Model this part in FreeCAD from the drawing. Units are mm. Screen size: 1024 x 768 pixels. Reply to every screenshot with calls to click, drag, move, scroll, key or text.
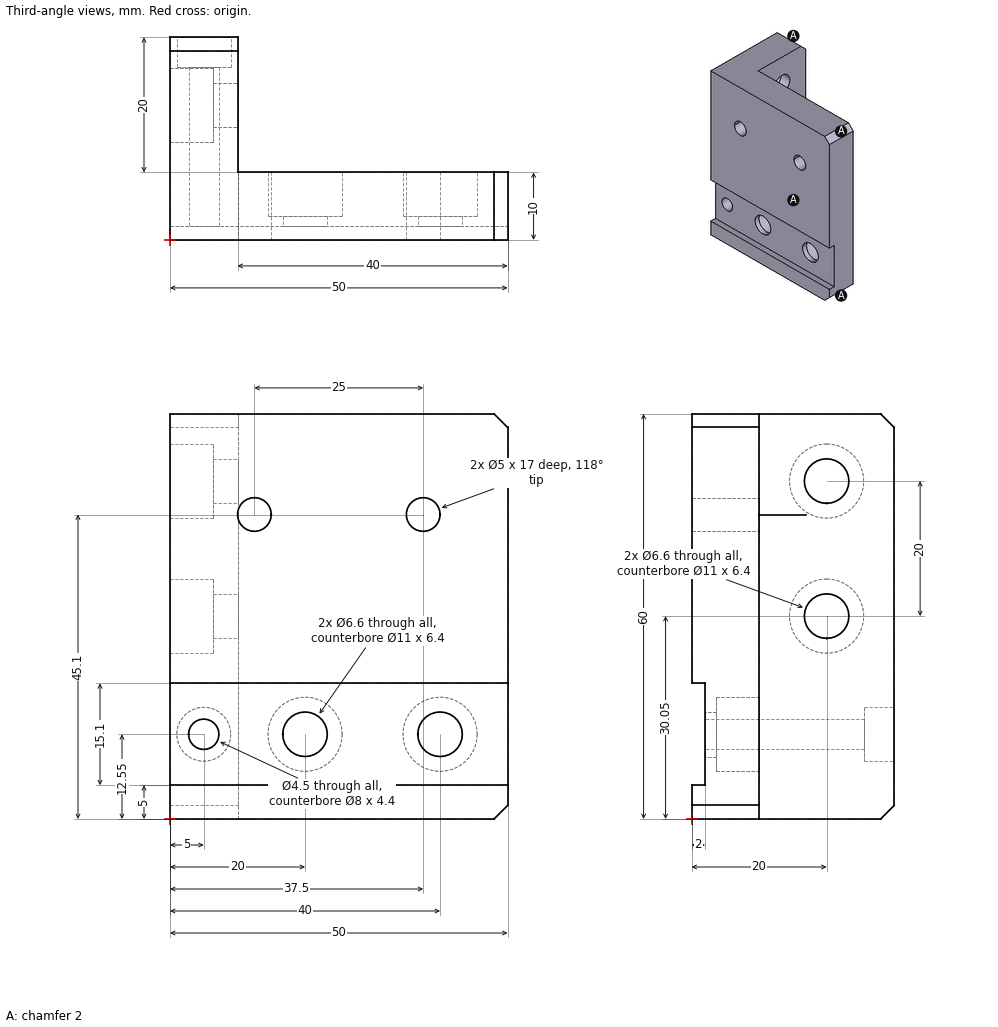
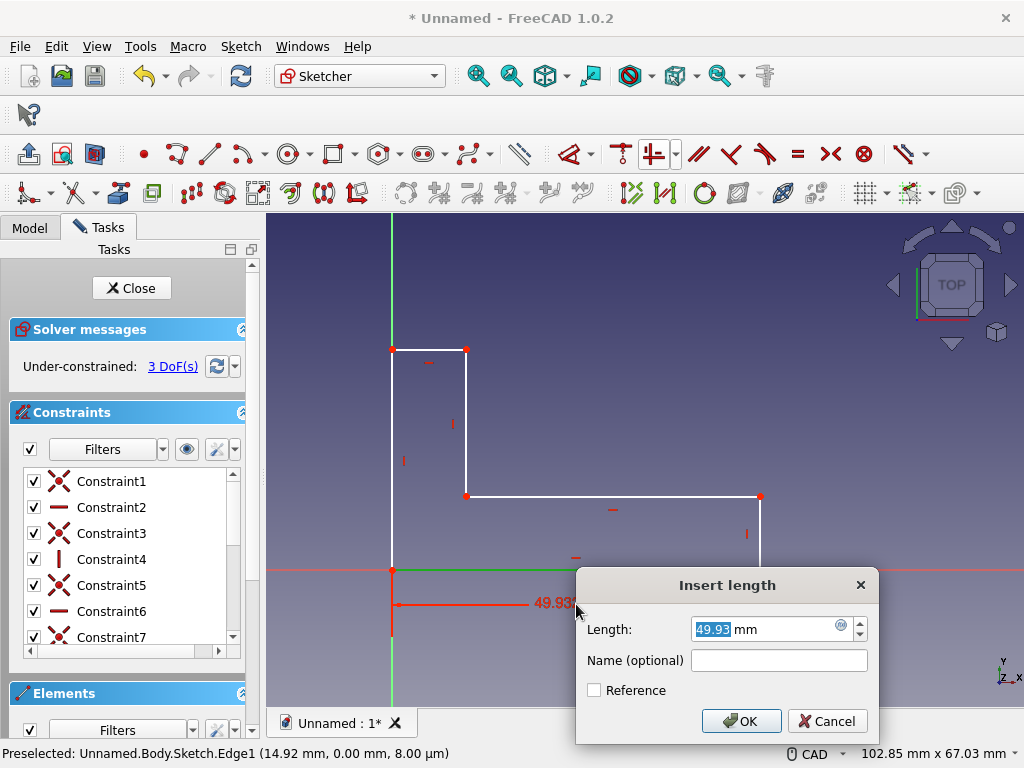
text(50)
key(Return)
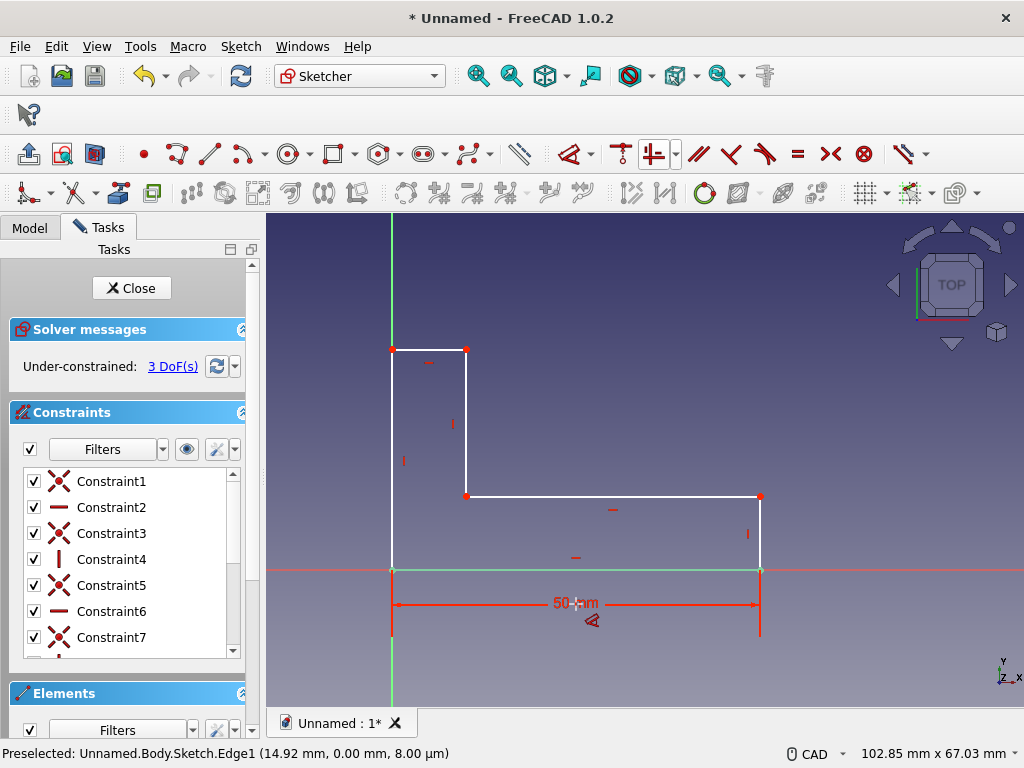
click(760, 548)
click(794, 534)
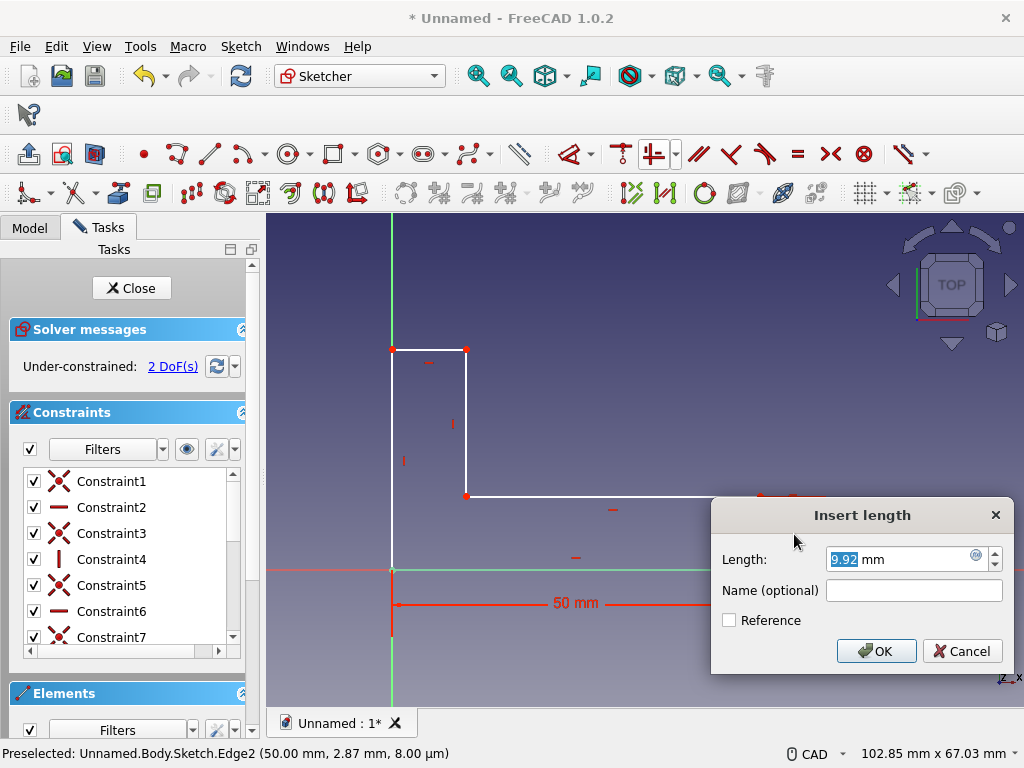
text(10)
key(Return)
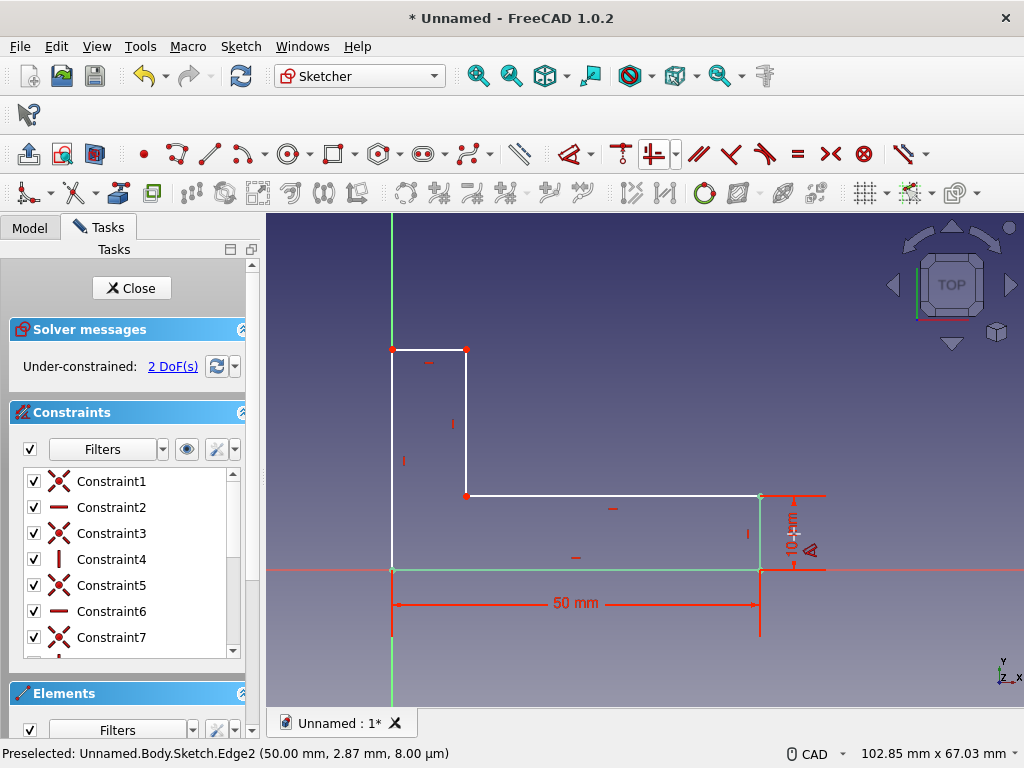
click(672, 496)
click(613, 530)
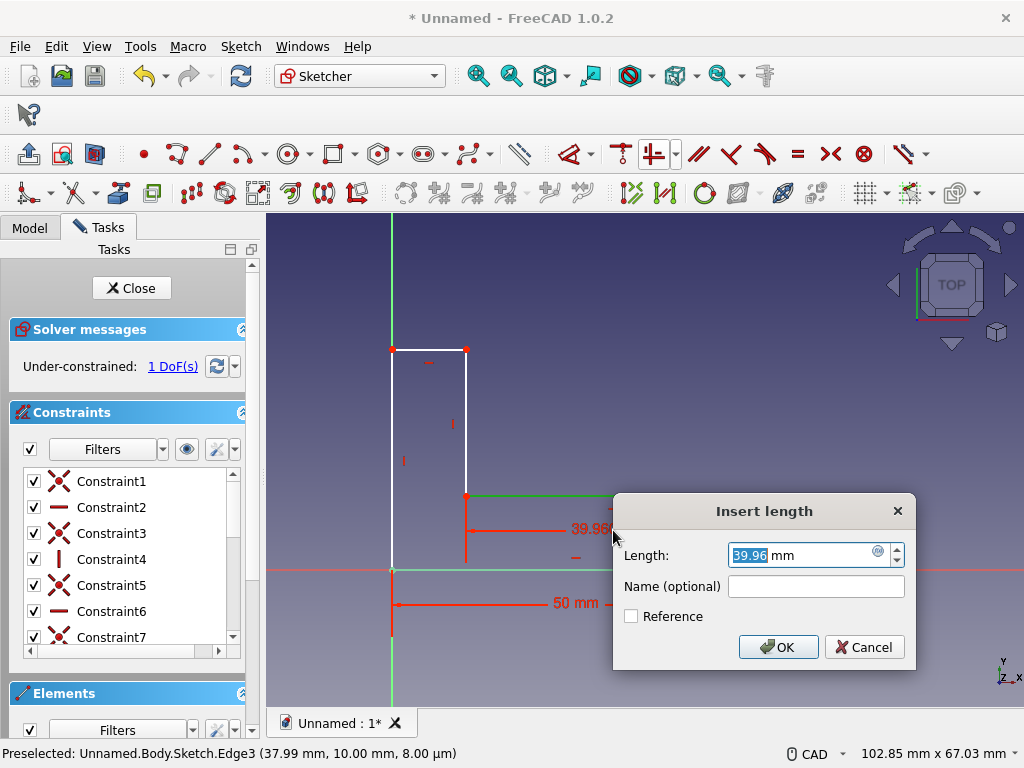
text(40)
key(Return)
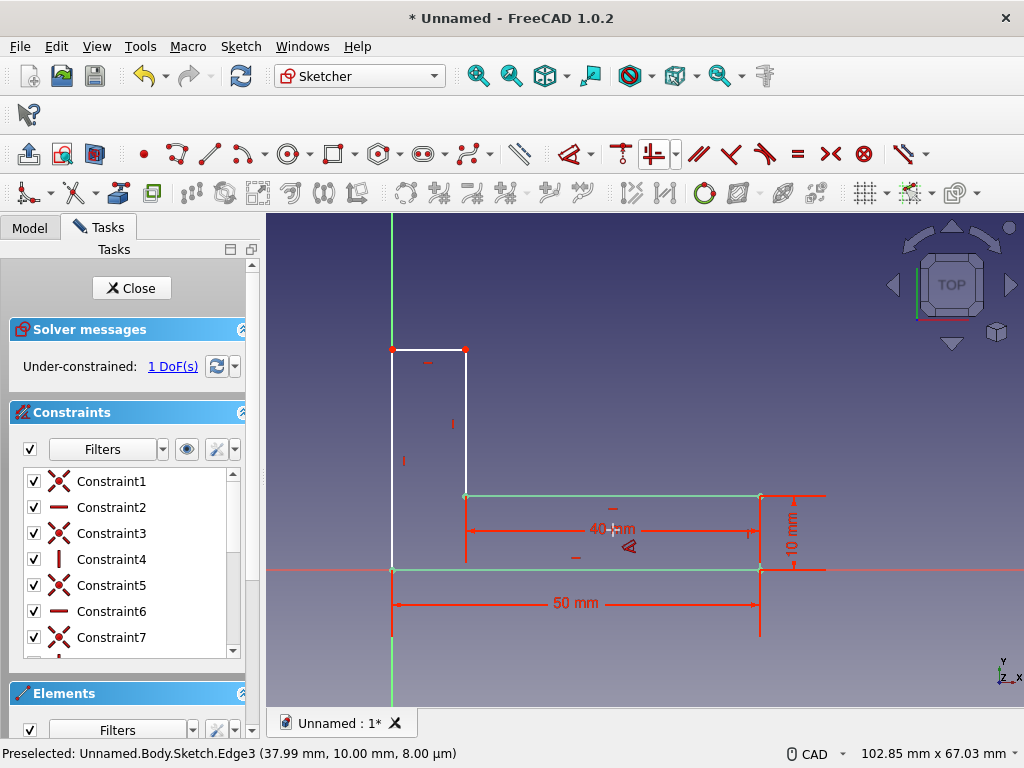
click(466, 453)
click(432, 423)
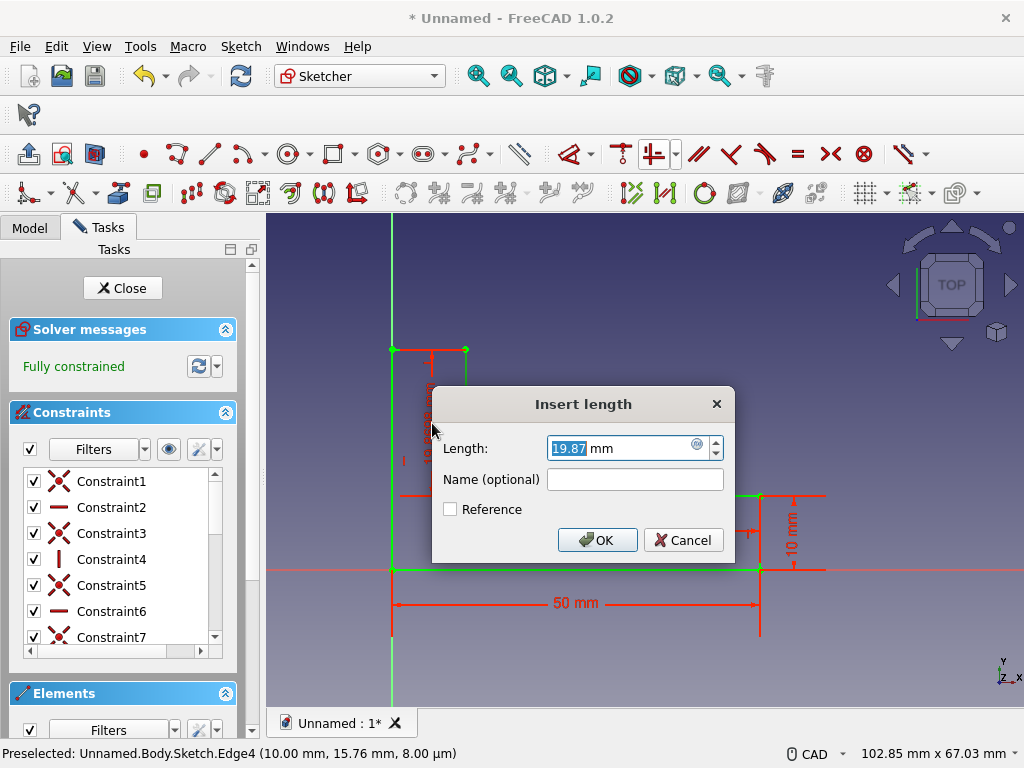
text(20)
key(Return)
key(Escape)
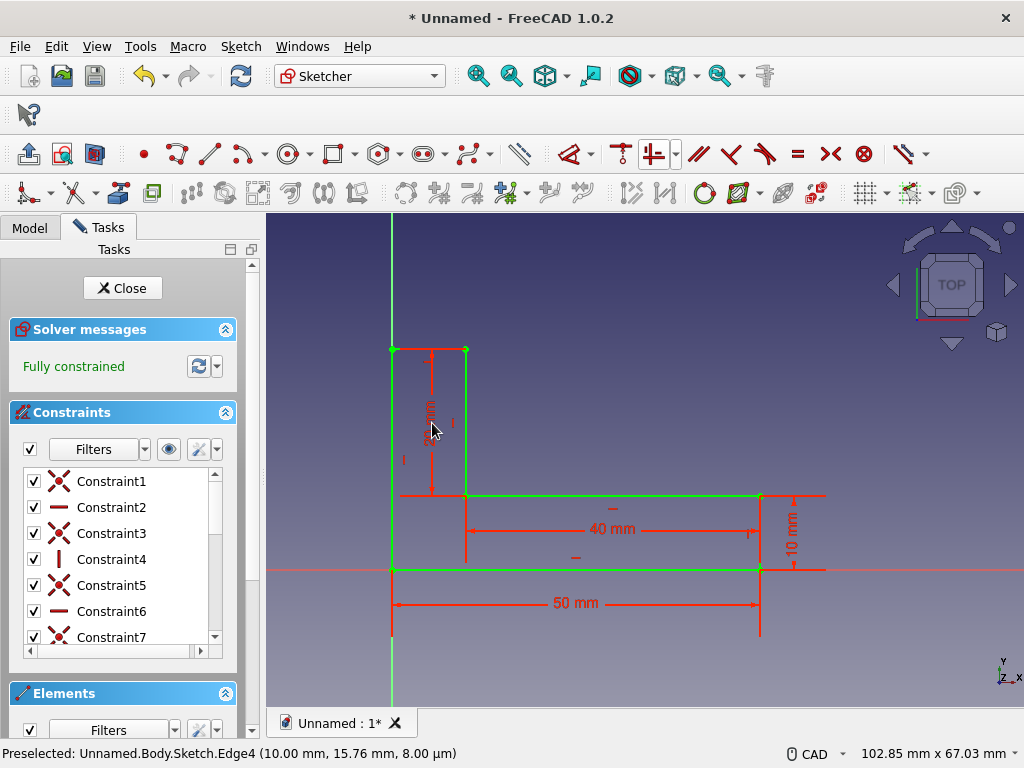
click(123, 288)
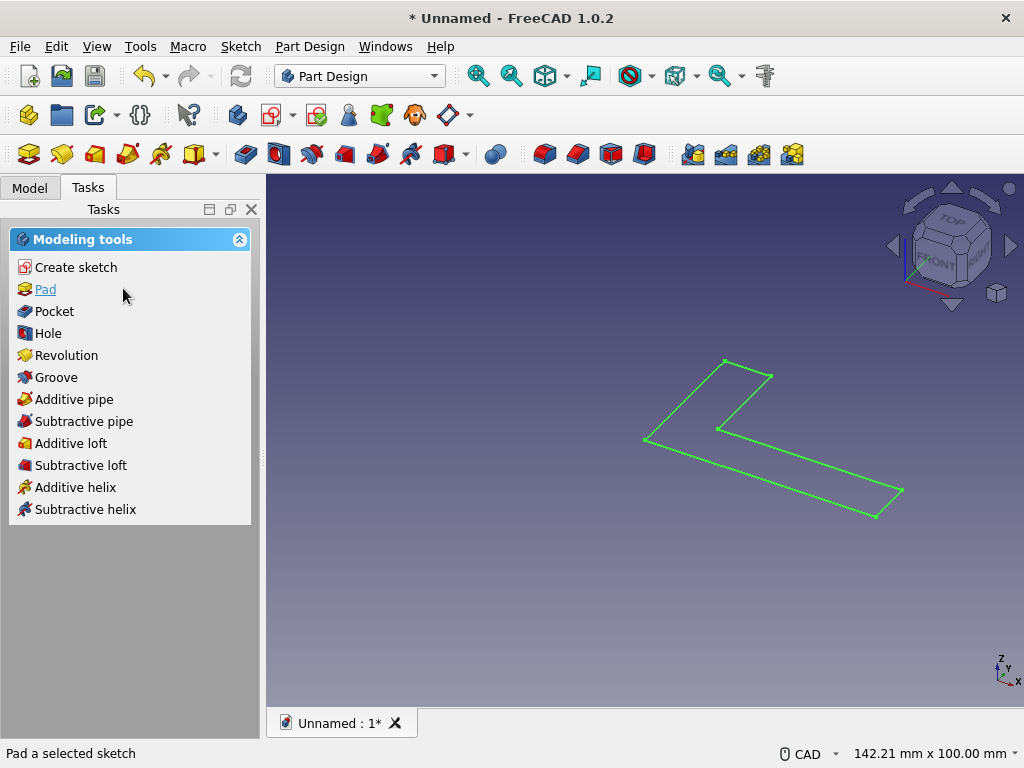
click(29, 154)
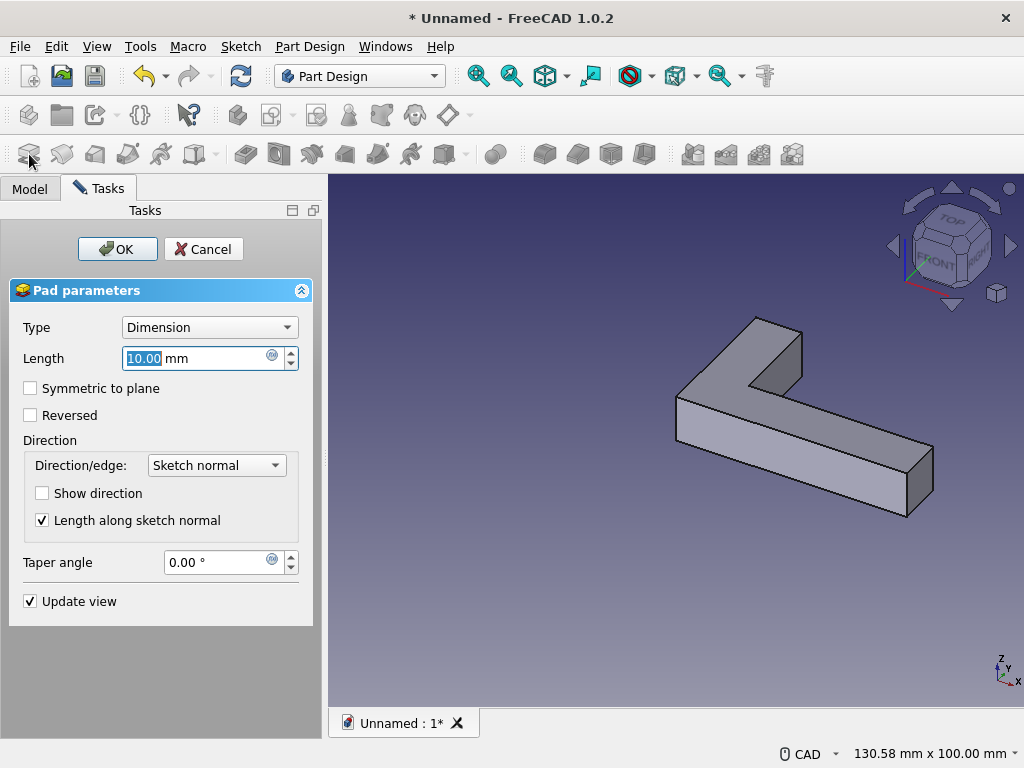
text(60)
key(Tab)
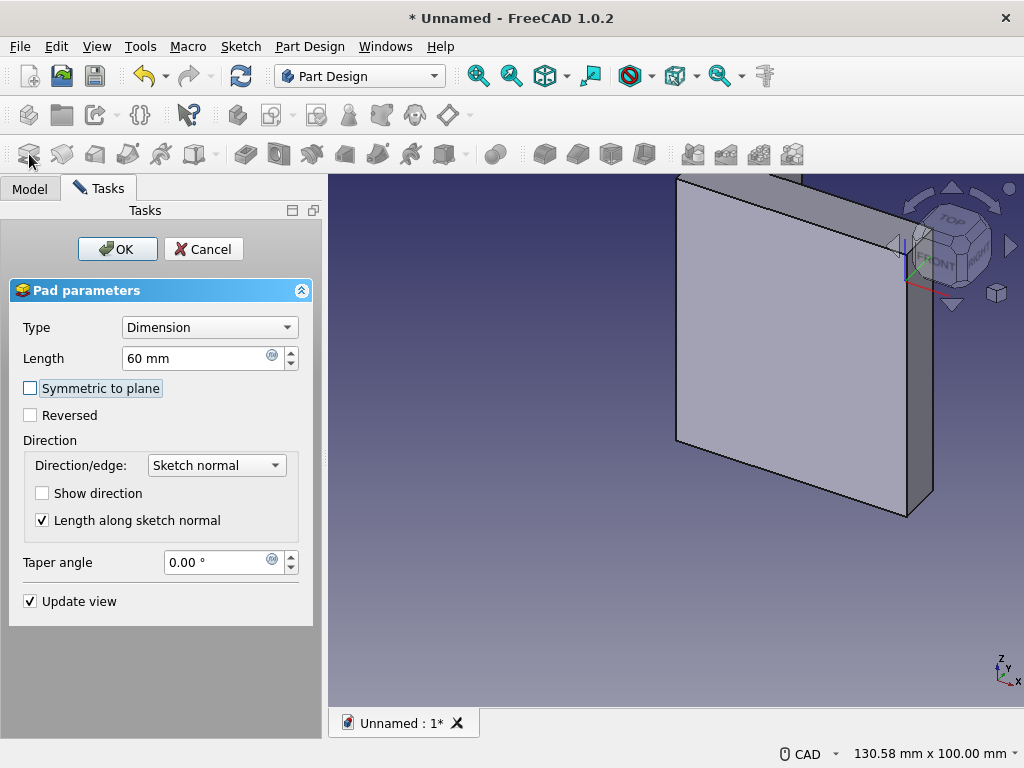
click(118, 249)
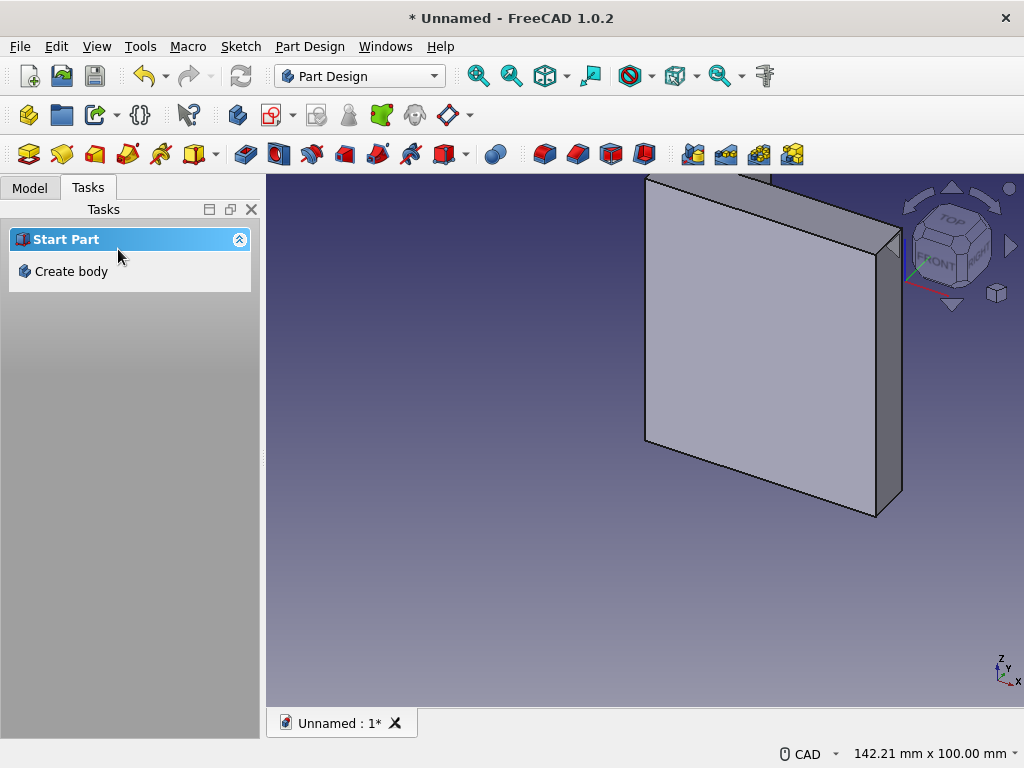
click(479, 76)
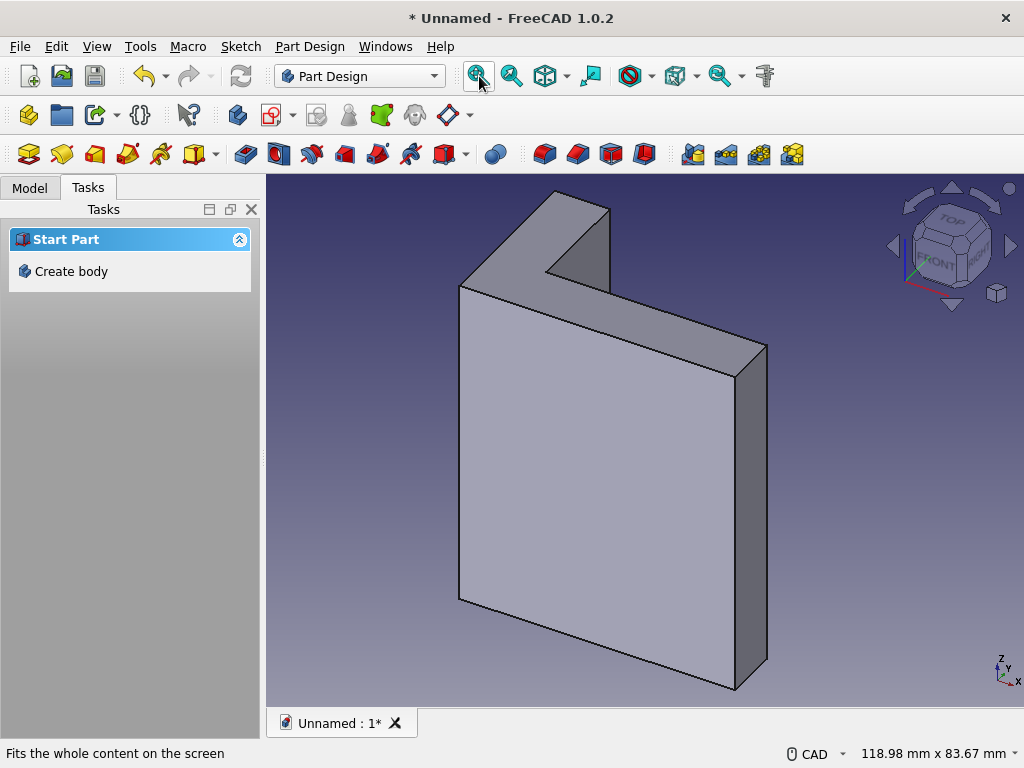
click(270, 116)